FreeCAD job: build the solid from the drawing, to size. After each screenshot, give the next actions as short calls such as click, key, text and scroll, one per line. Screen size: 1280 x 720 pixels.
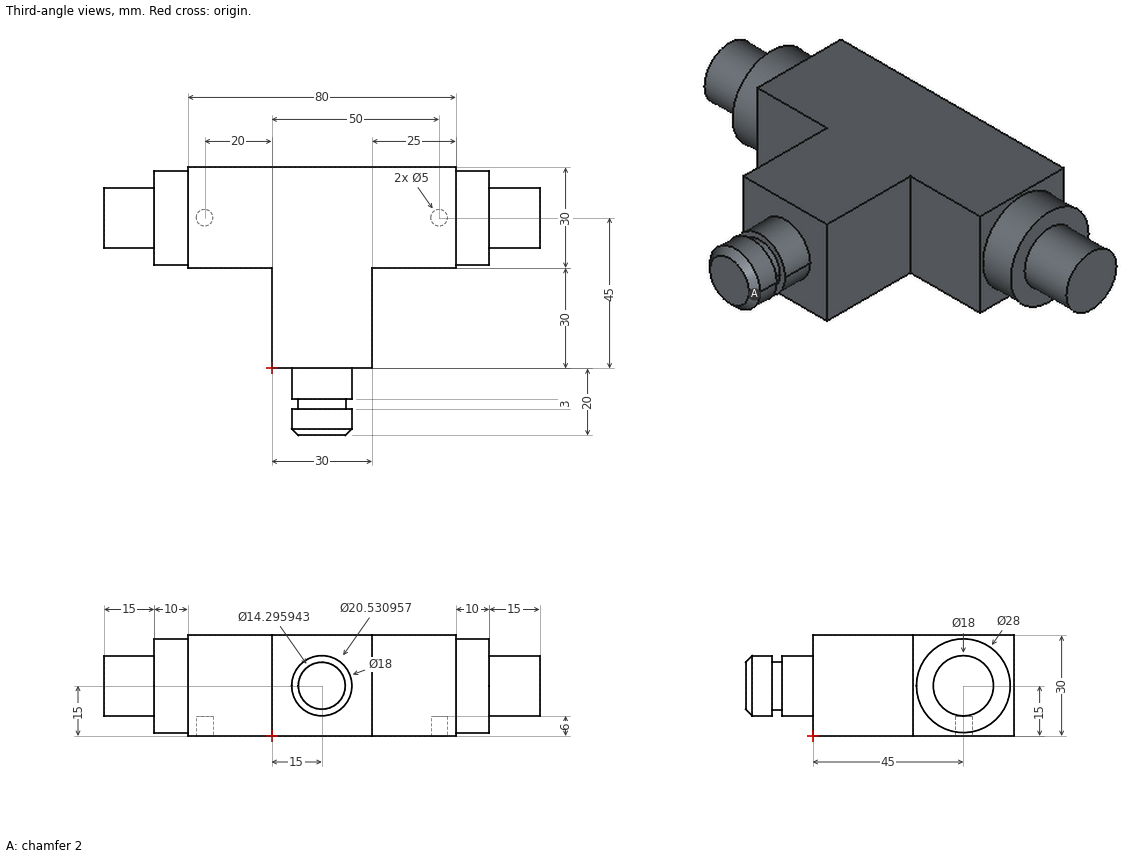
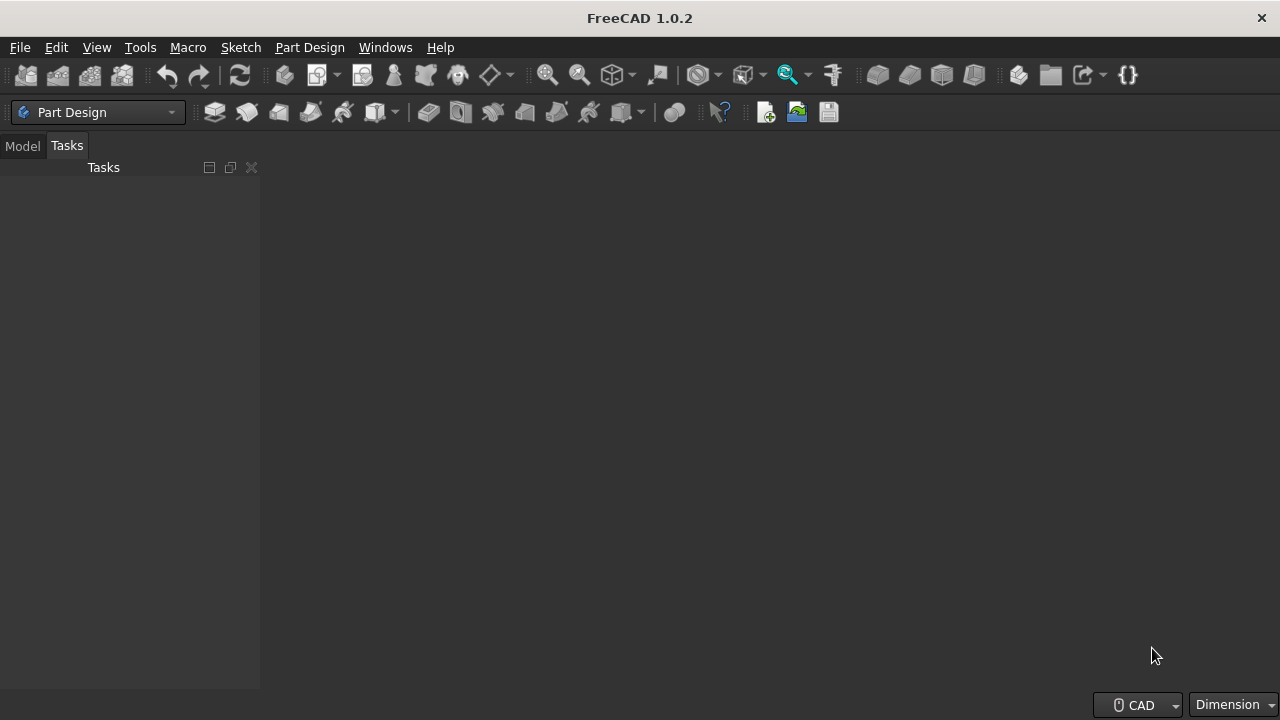
key(ctrl+n)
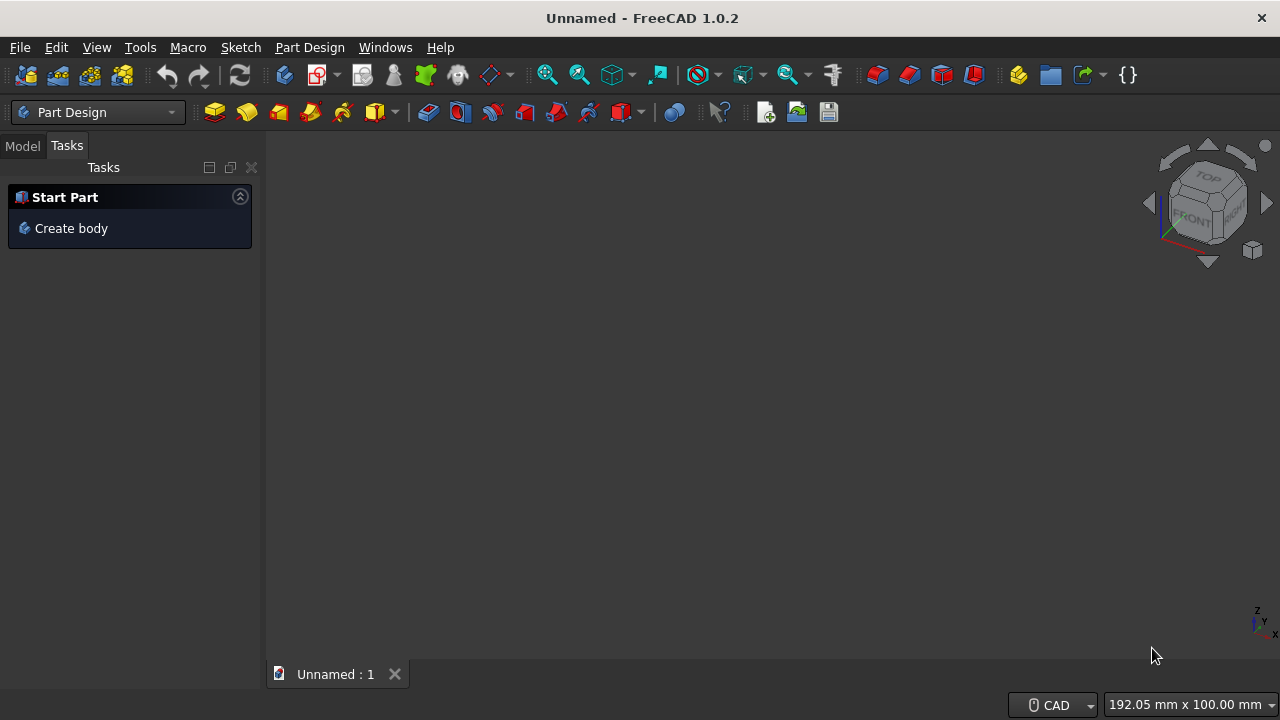
click(318, 76)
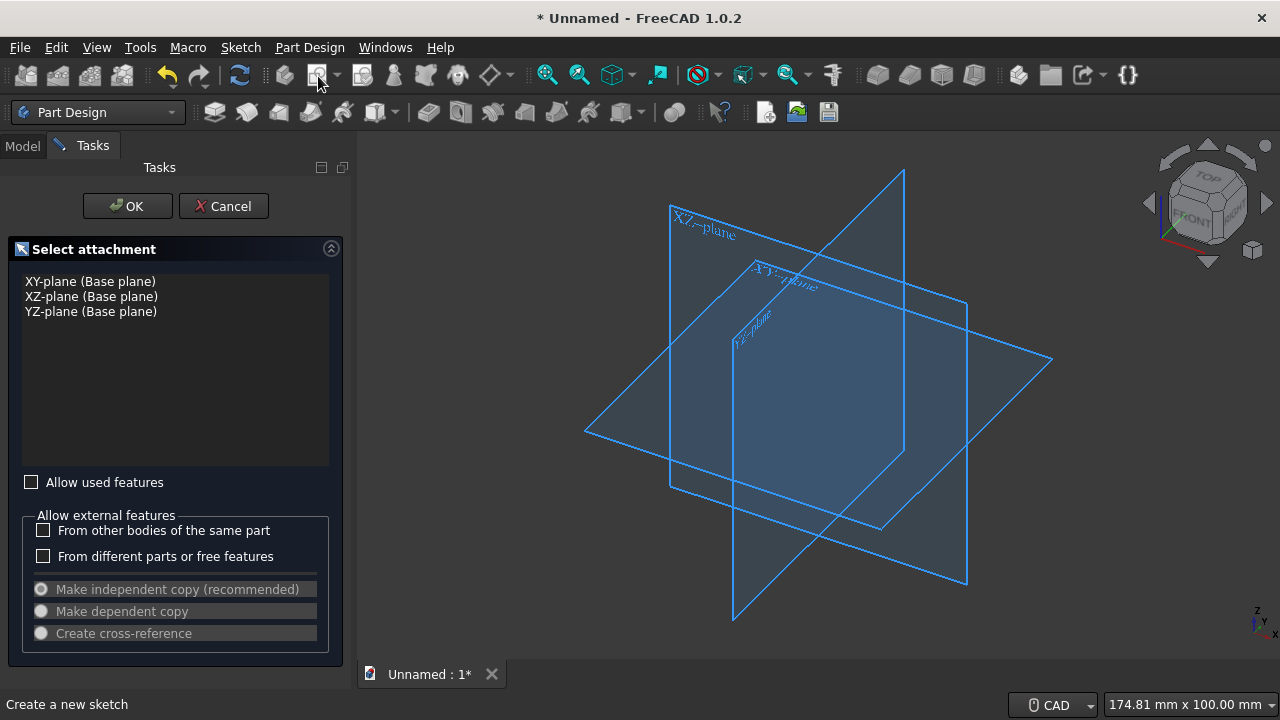
click(82, 282)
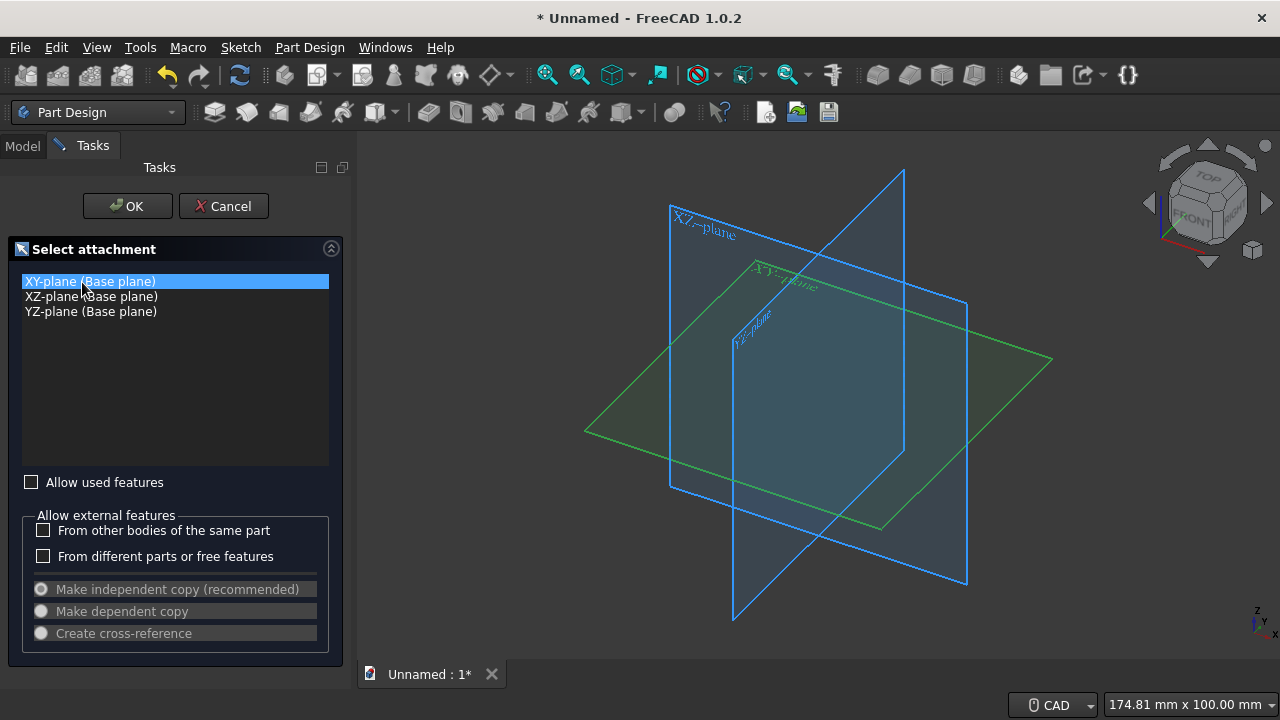
click(128, 206)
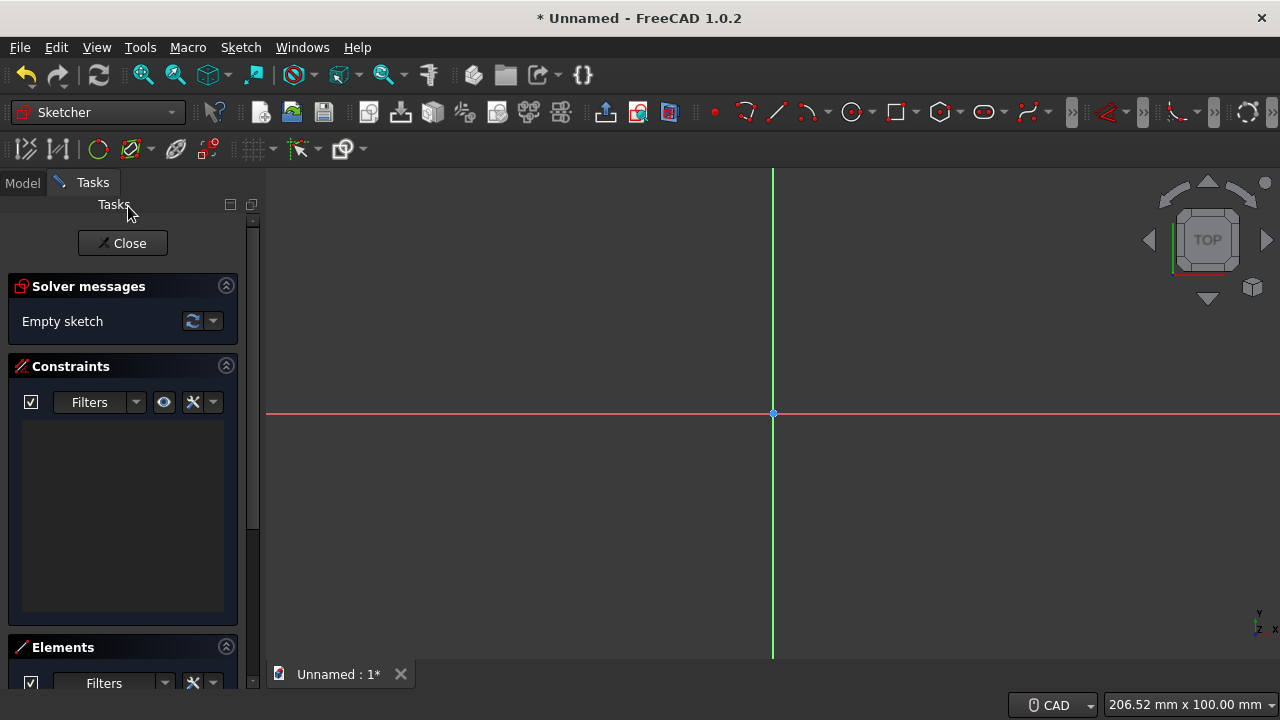
scroll(415, 631, down, 2)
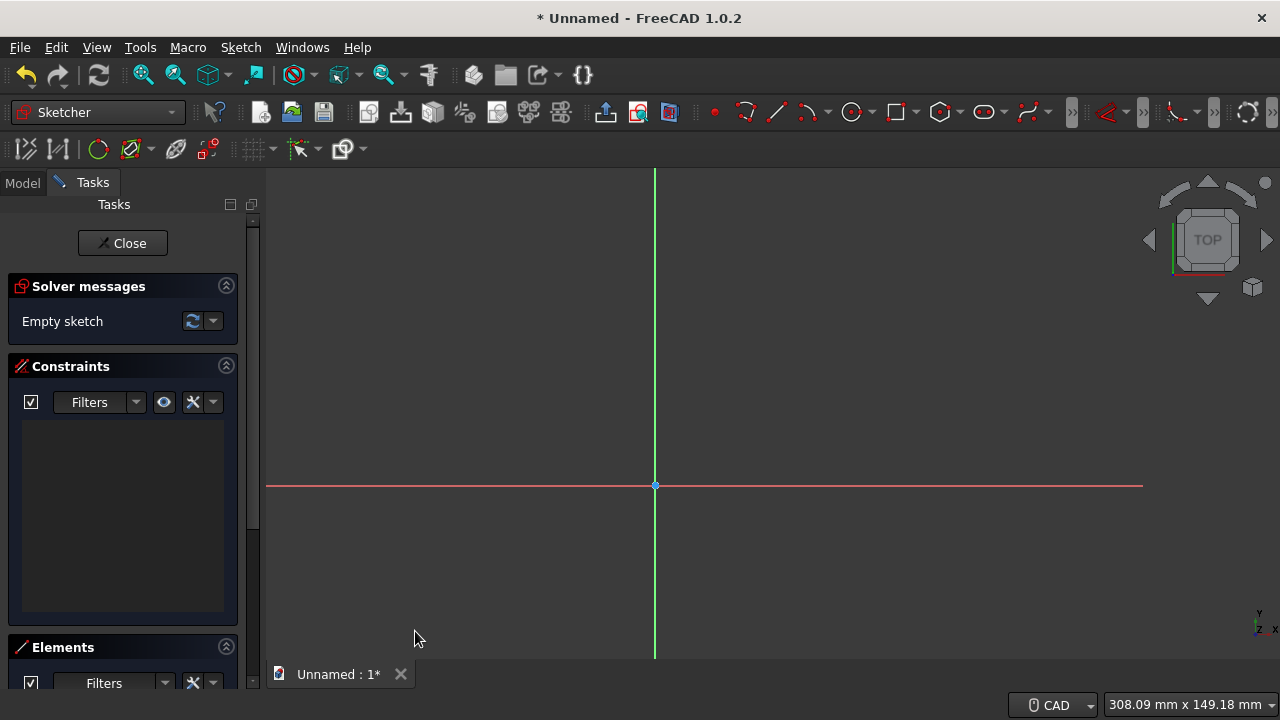
scroll(704, 332, up, 2)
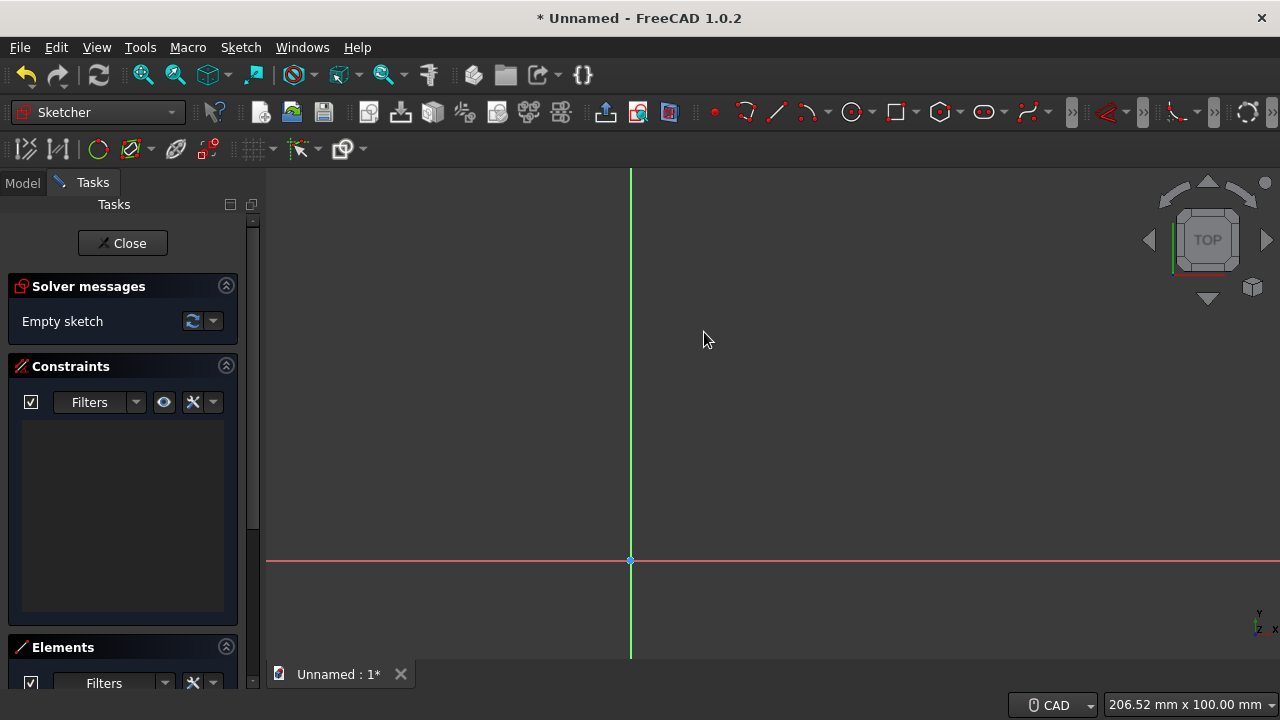
click(746, 112)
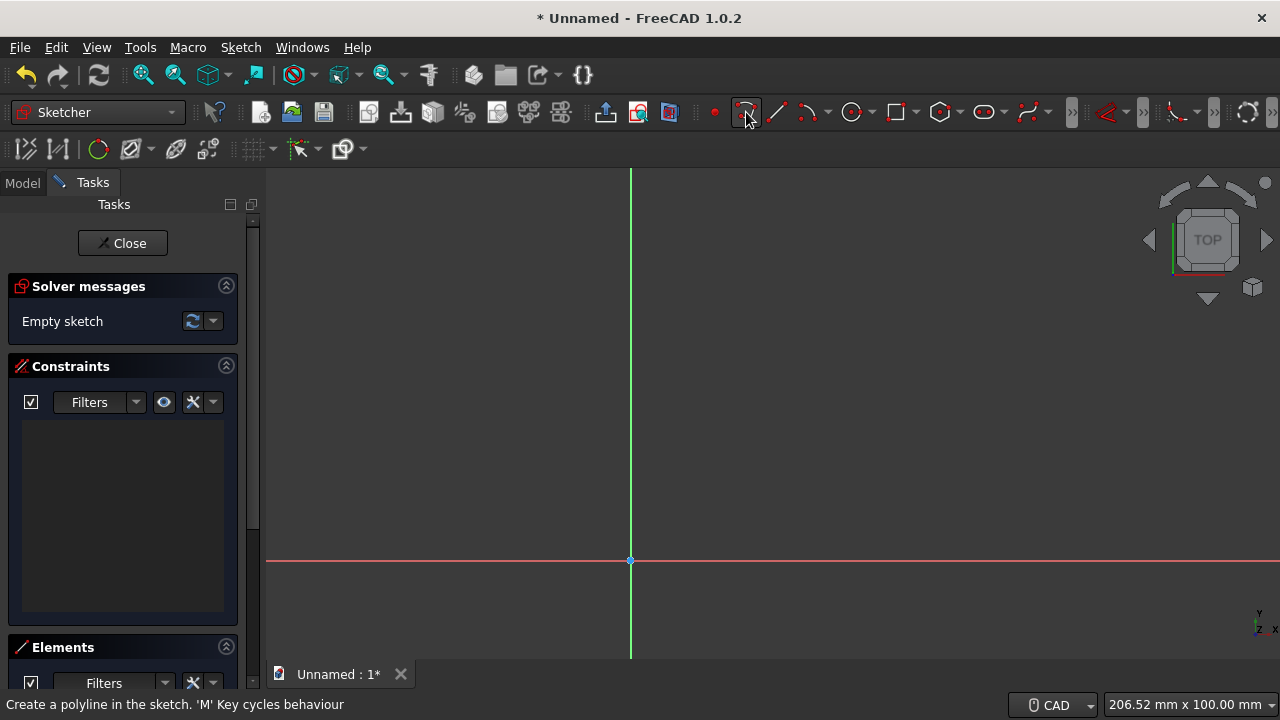
click(631, 561)
click(778, 552)
click(778, 414)
click(901, 414)
click(901, 266)
click(508, 266)
click(508, 414)
click(640, 414)
click(631, 561)
key(Escape)
key(Escape)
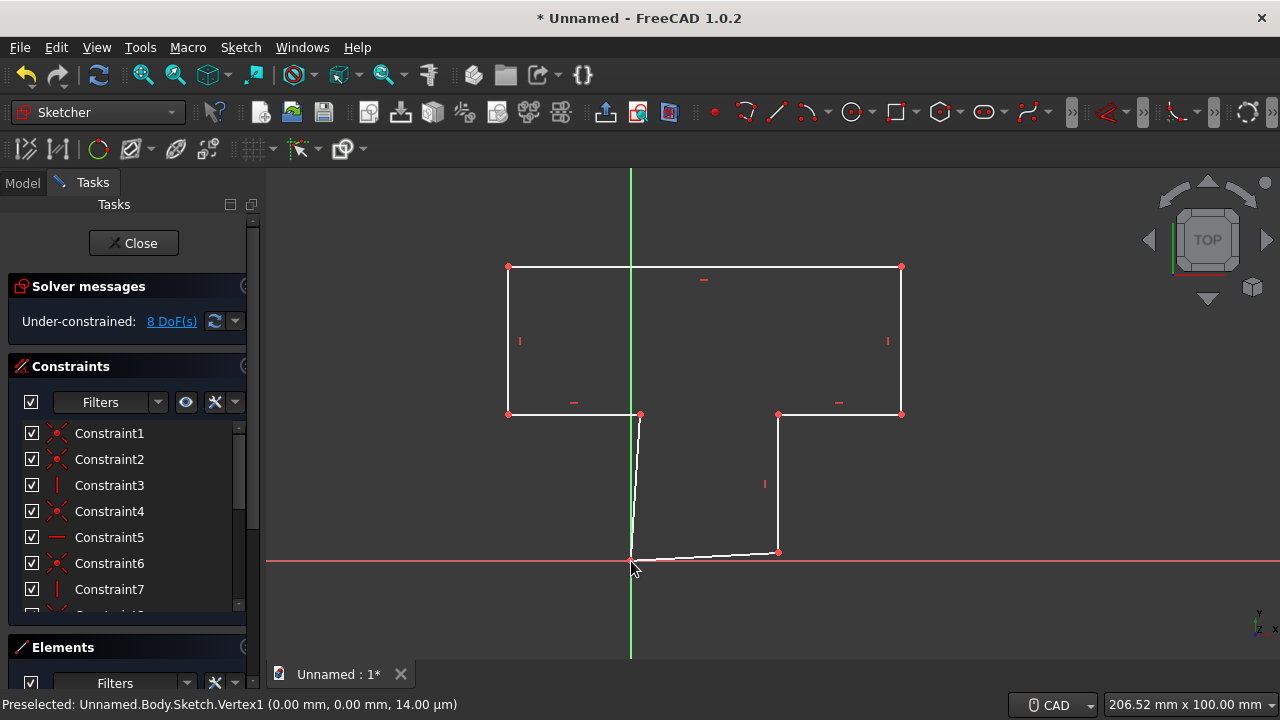
click(675, 558)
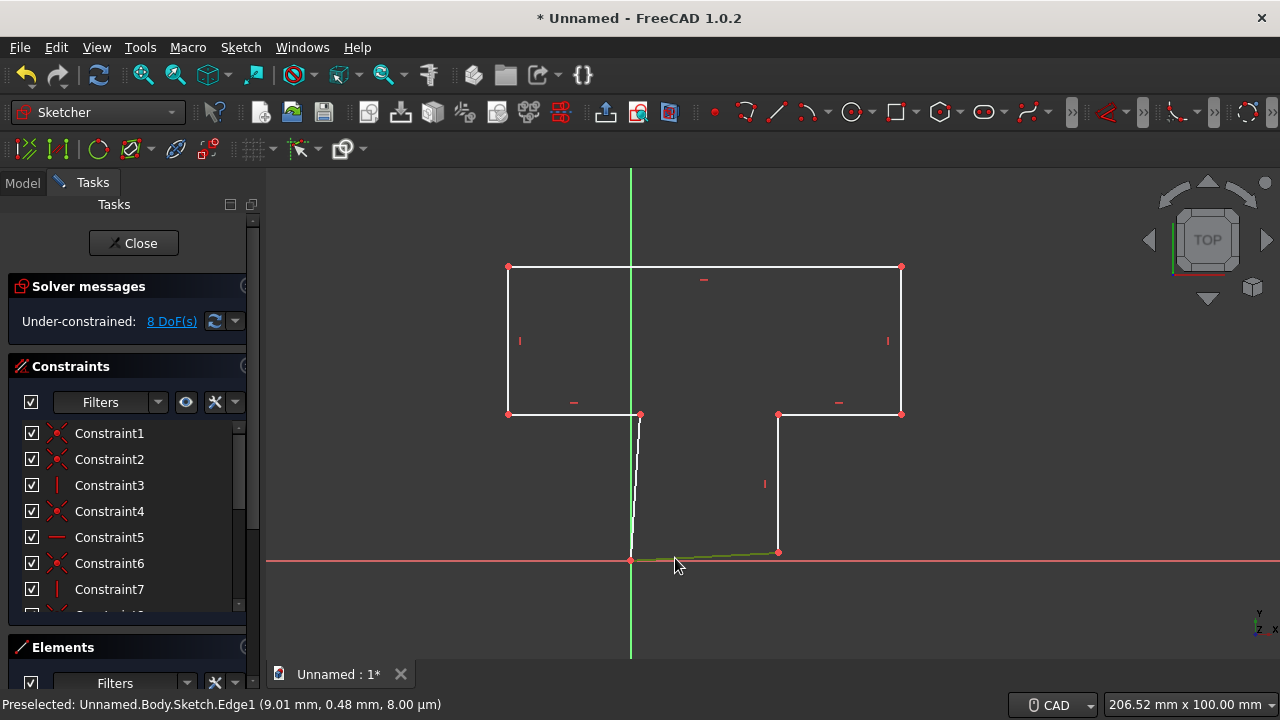
key(h)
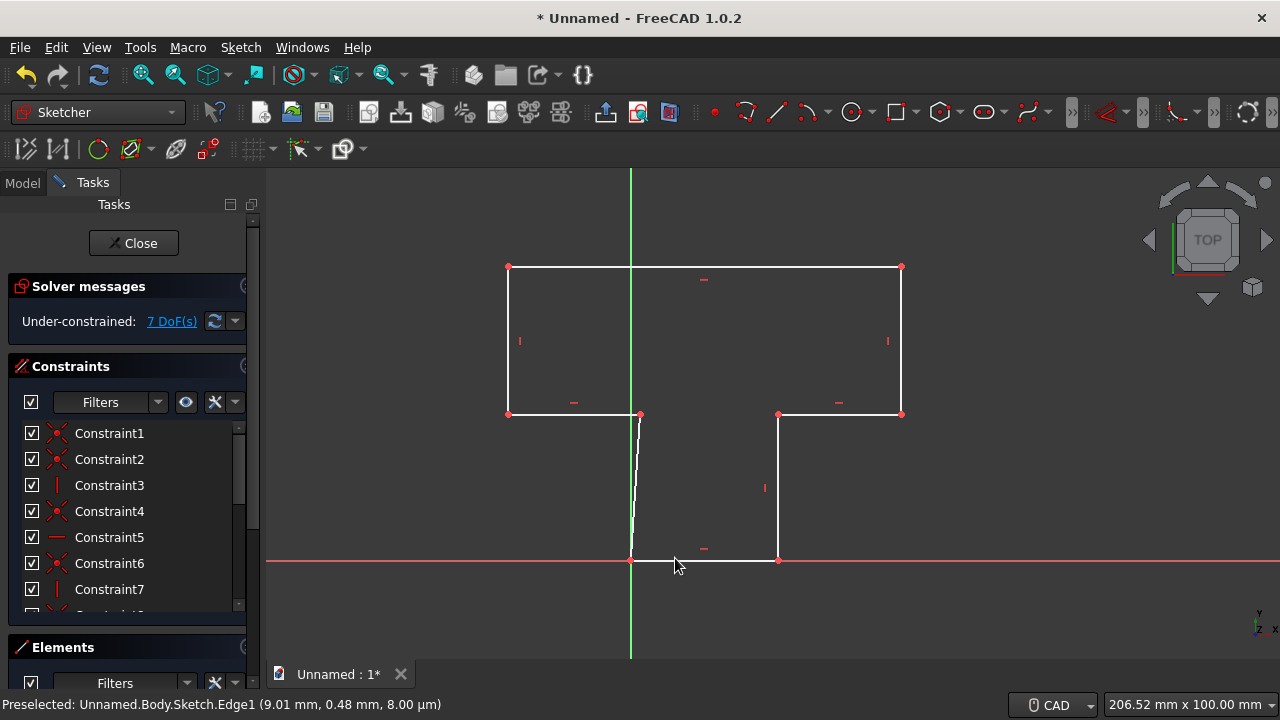
click(634, 517)